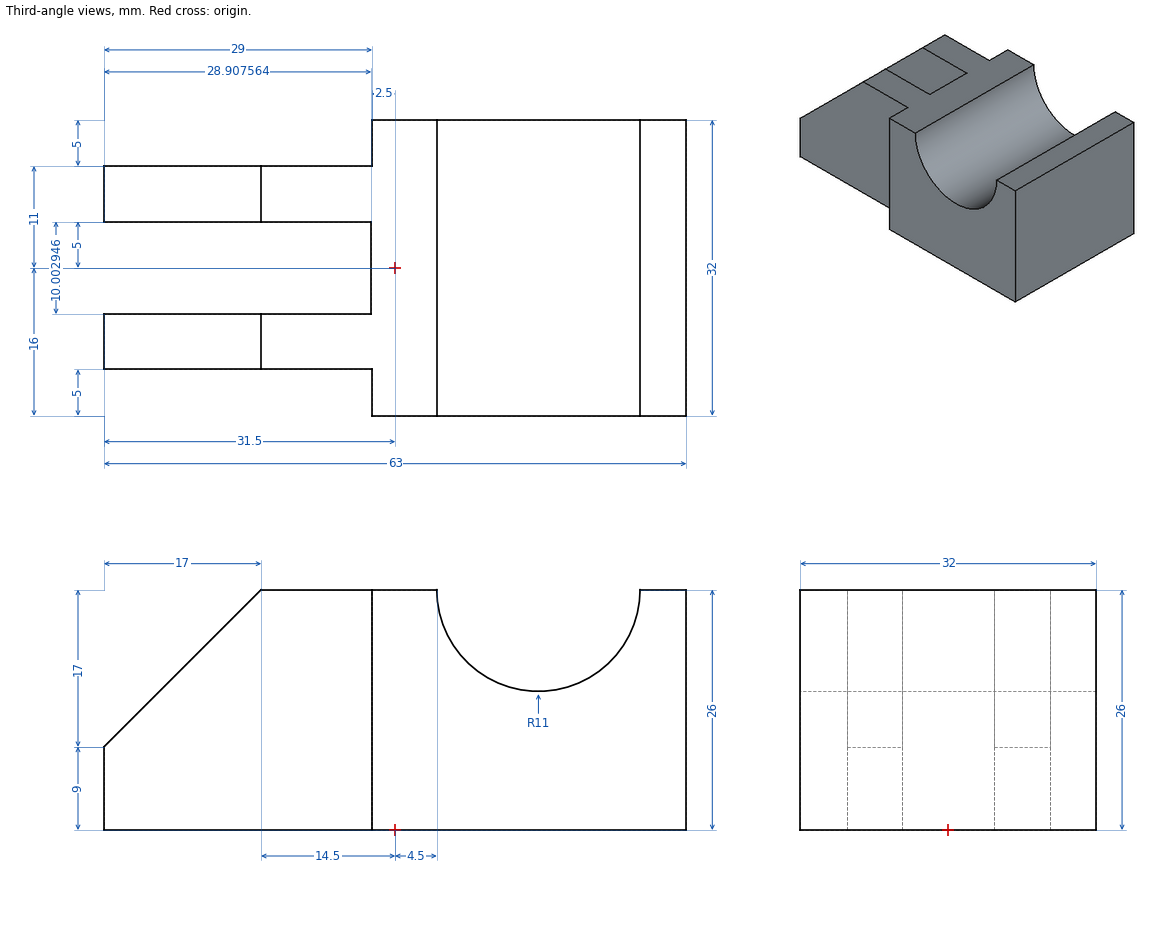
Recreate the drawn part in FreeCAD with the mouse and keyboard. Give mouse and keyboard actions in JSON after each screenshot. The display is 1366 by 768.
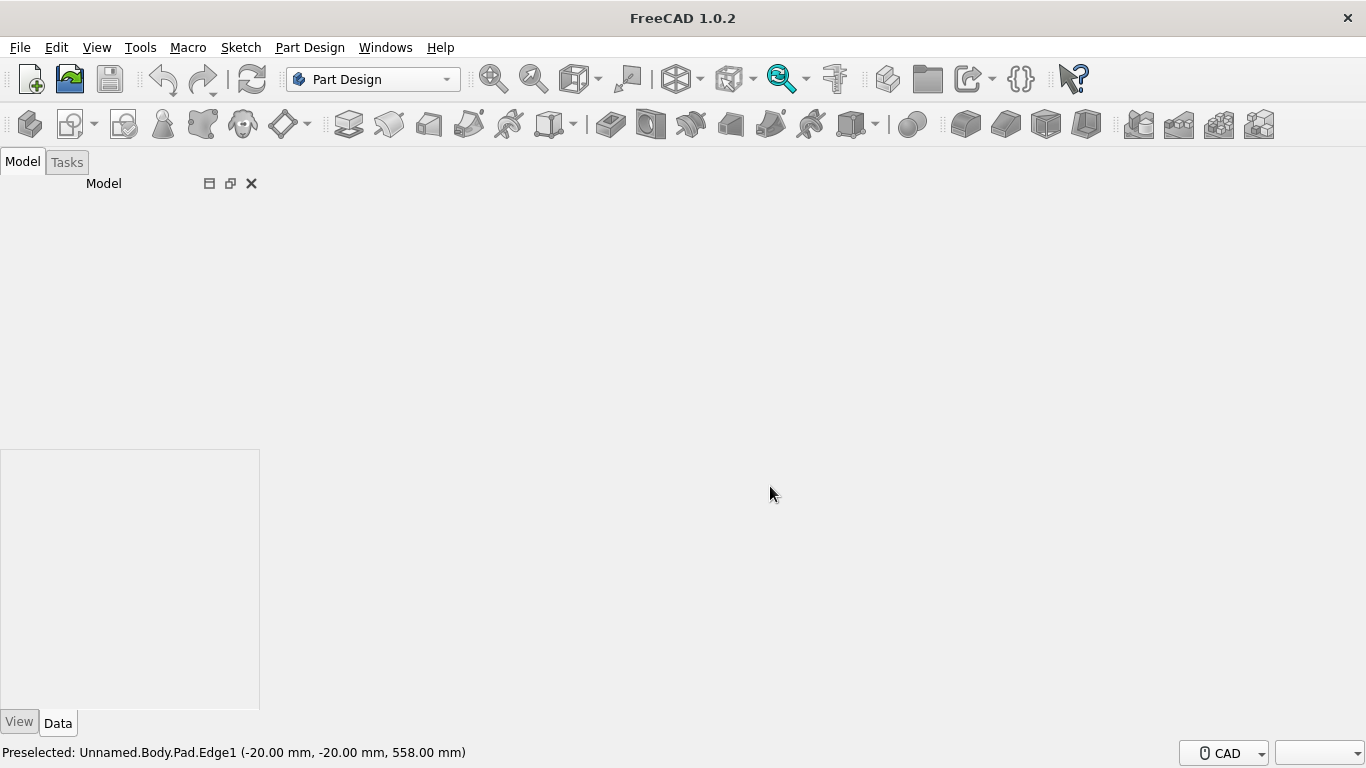
{"action": "left_click", "coordinate": [30, 80]}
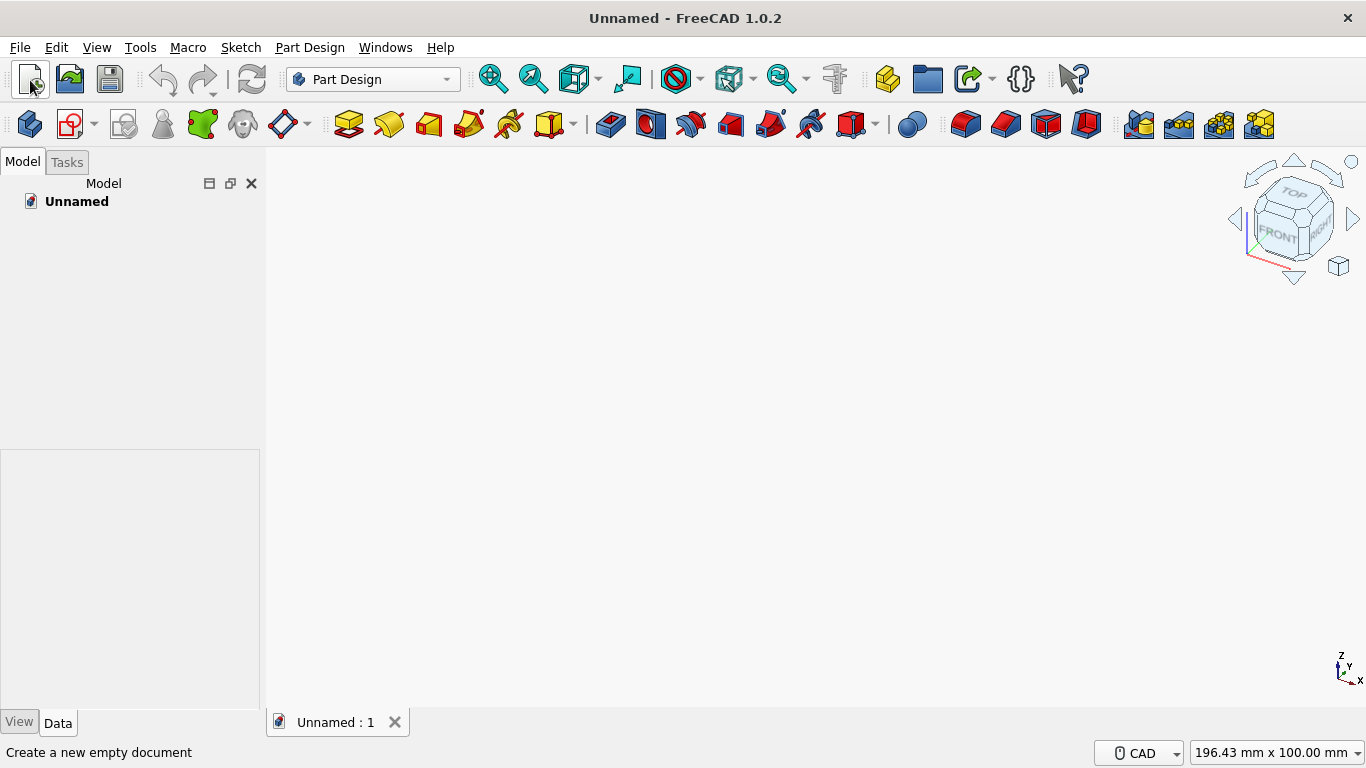
{"action": "left_click", "coordinate": [70, 124]}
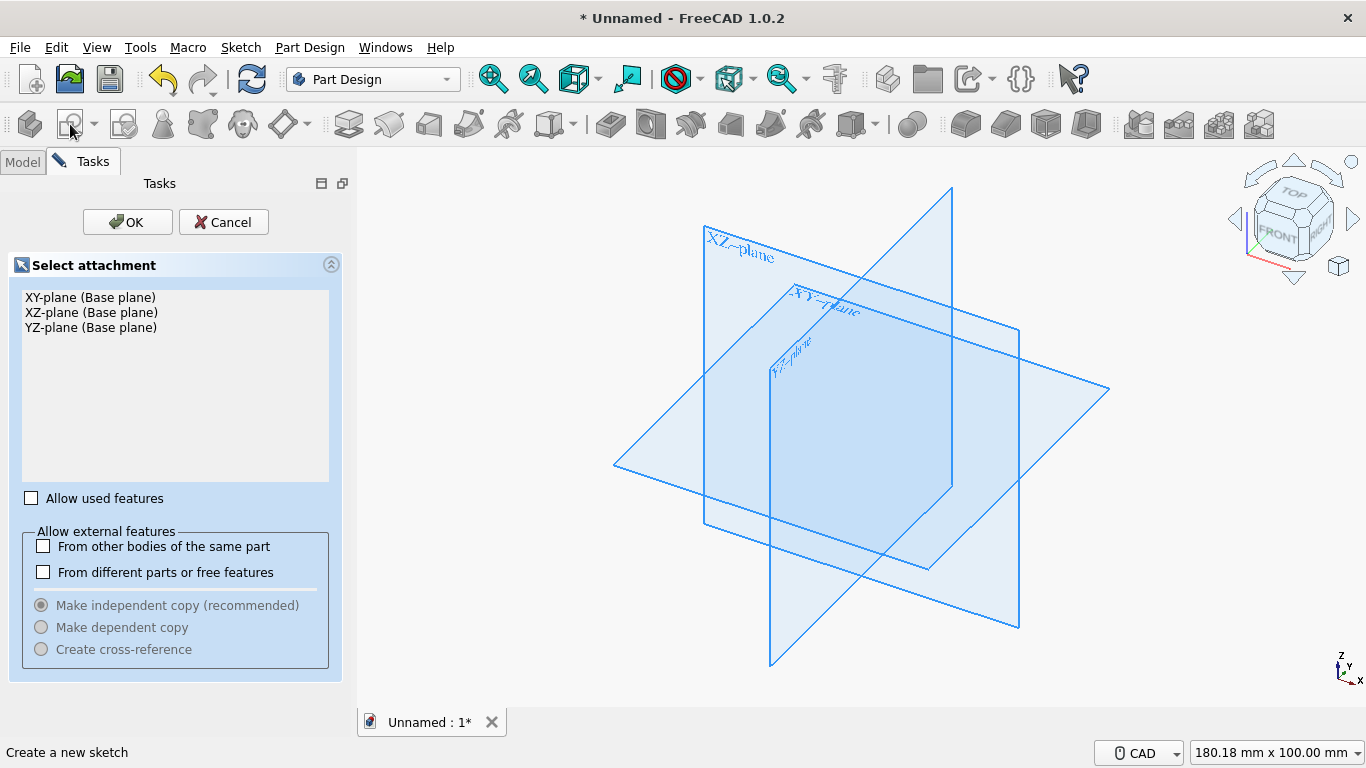
{"action": "left_click", "coordinate": [82, 298]}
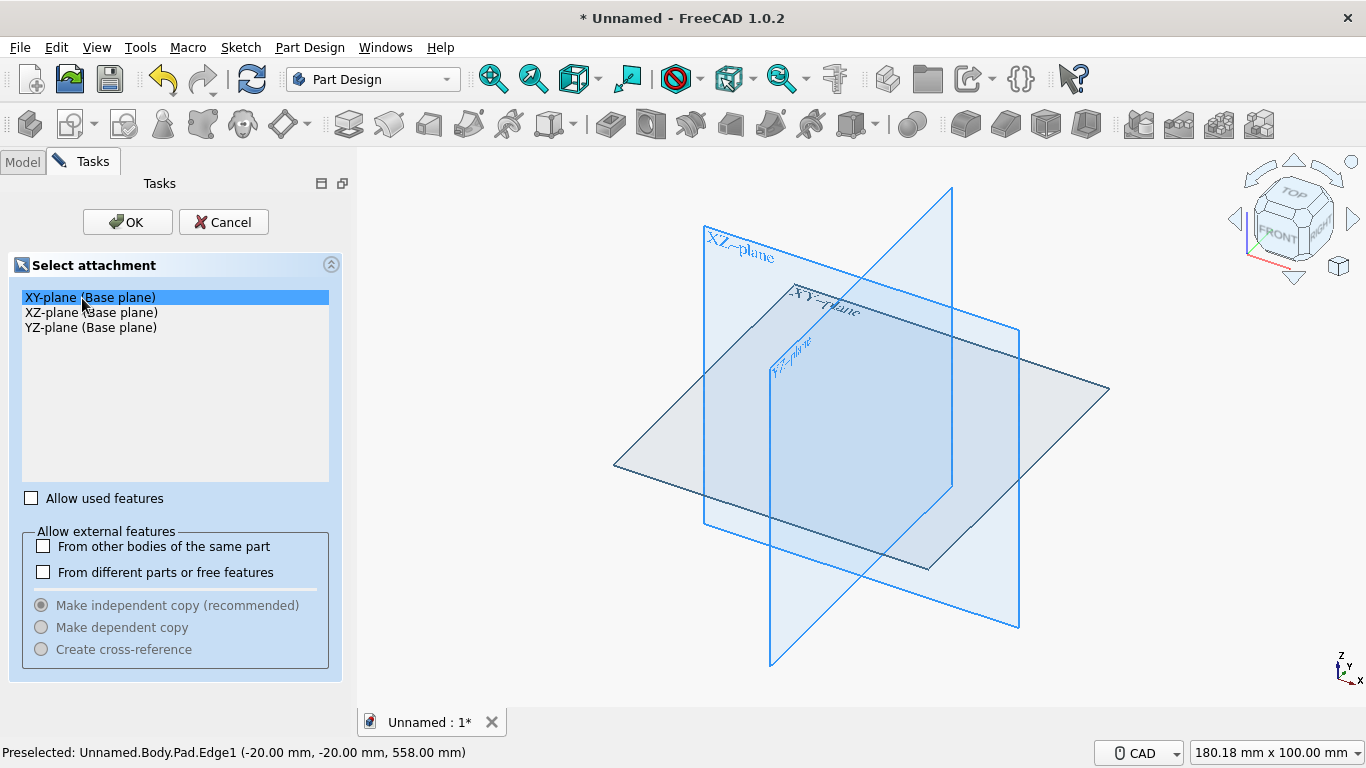
{"action": "left_click", "coordinate": [128, 222]}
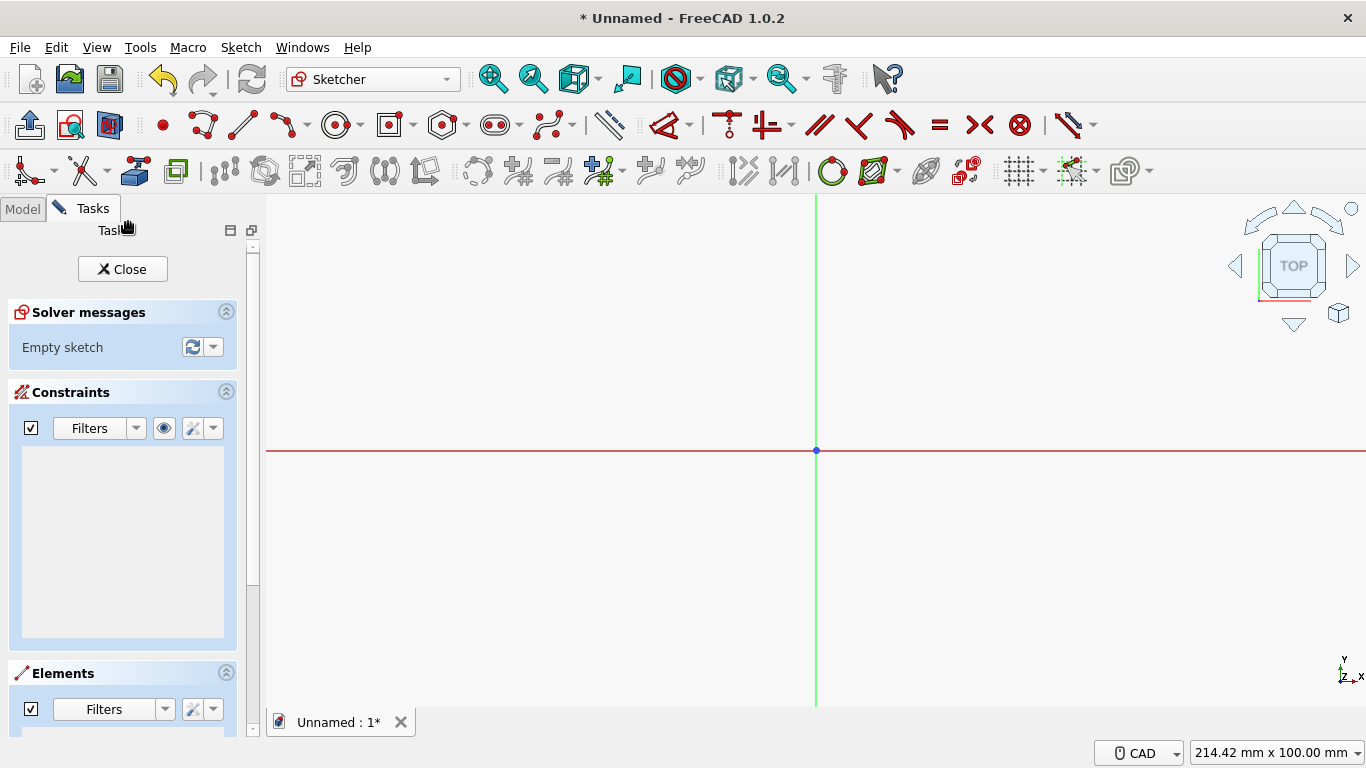
{"action": "scroll", "coordinate": [899, 450], "scroll_direction": "up", "scroll_amount": 3}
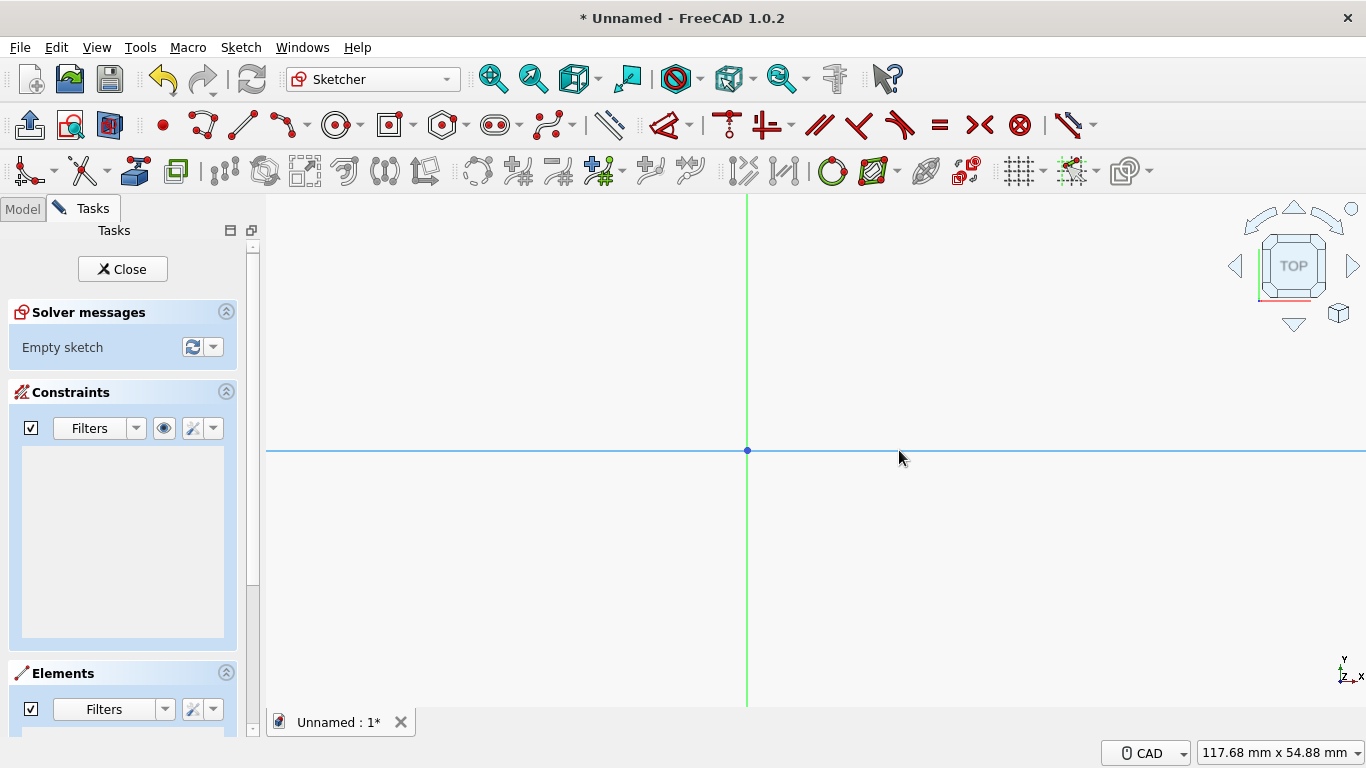
{"action": "left_click", "coordinate": [390, 126]}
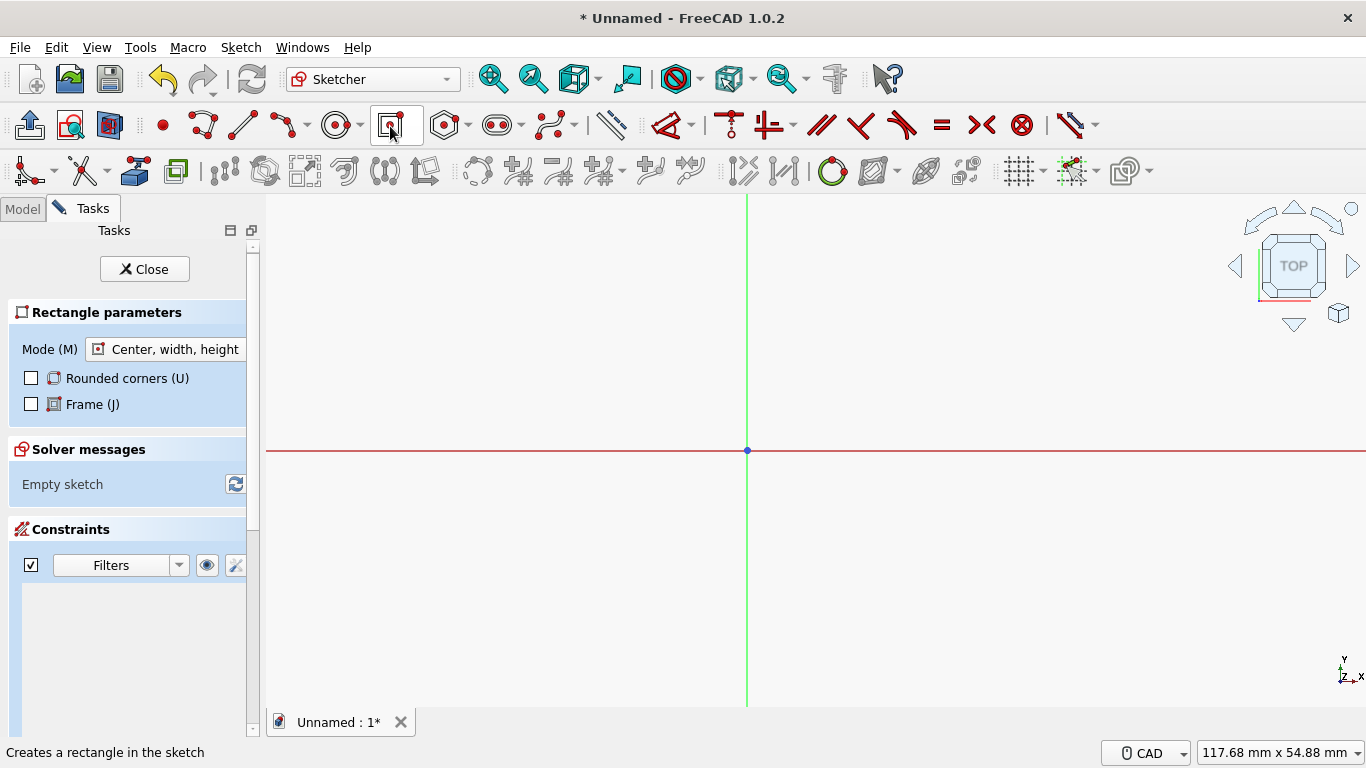
{"action": "left_click", "coordinate": [747, 450]}
{"action": "left_click", "coordinate": [1042, 301]}
{"action": "key", "text": "Escape"}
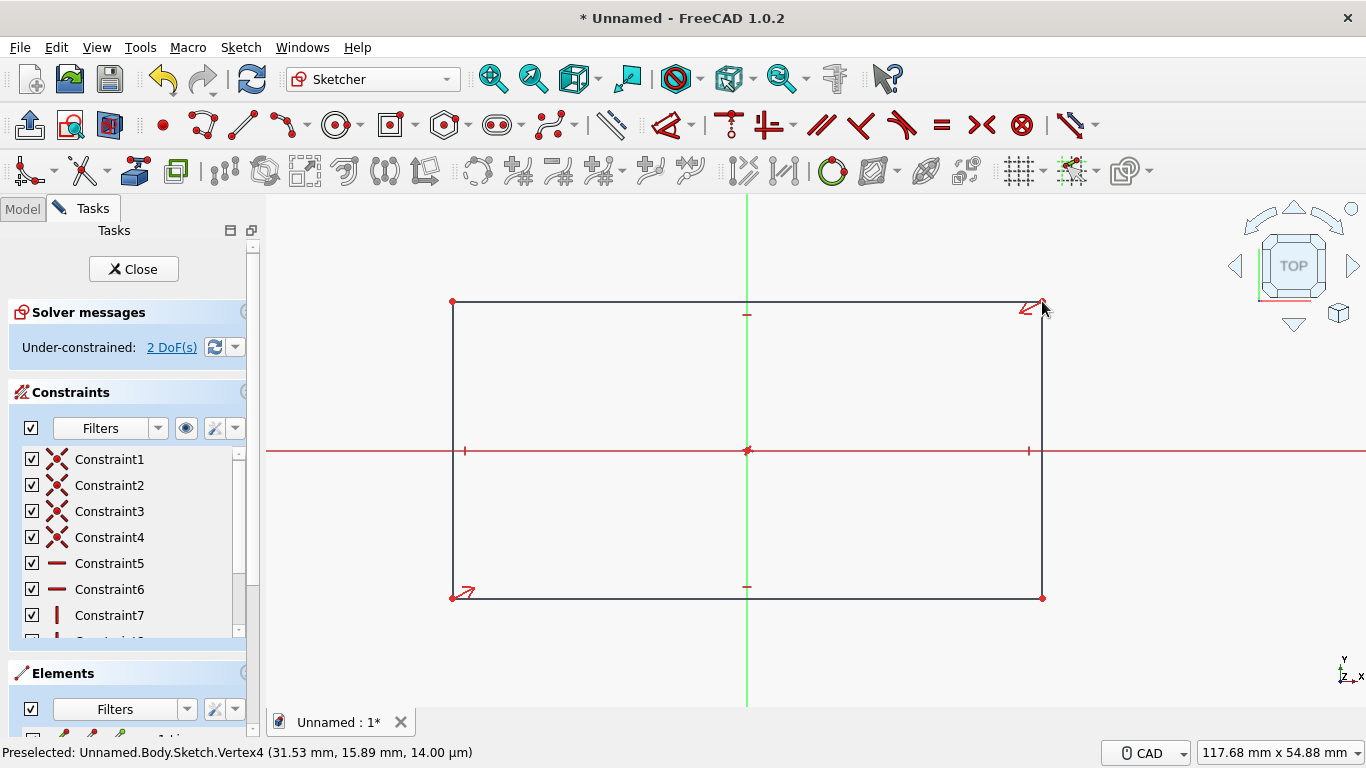
{"action": "left_click", "coordinate": [666, 126]}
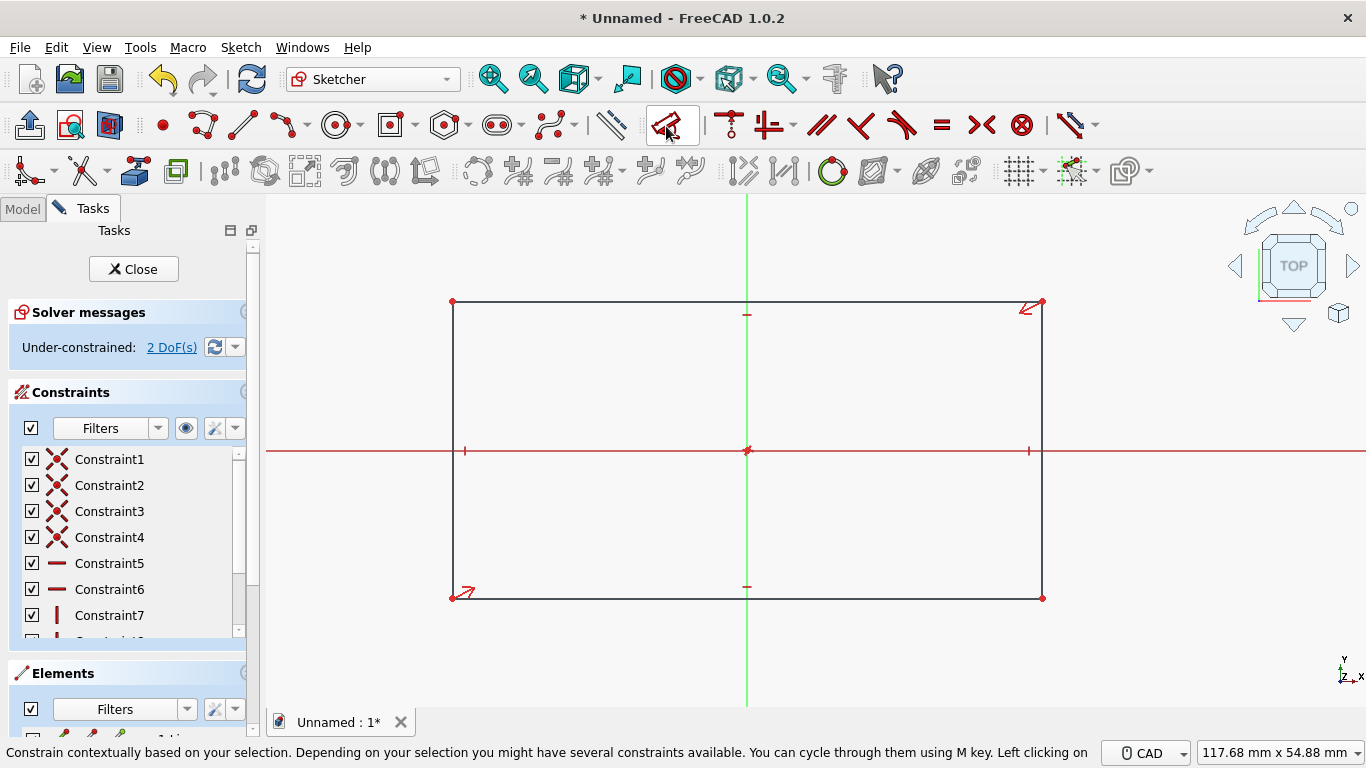
{"action": "left_click", "coordinate": [629, 599]}
{"action": "left_click", "coordinate": [612, 633]}